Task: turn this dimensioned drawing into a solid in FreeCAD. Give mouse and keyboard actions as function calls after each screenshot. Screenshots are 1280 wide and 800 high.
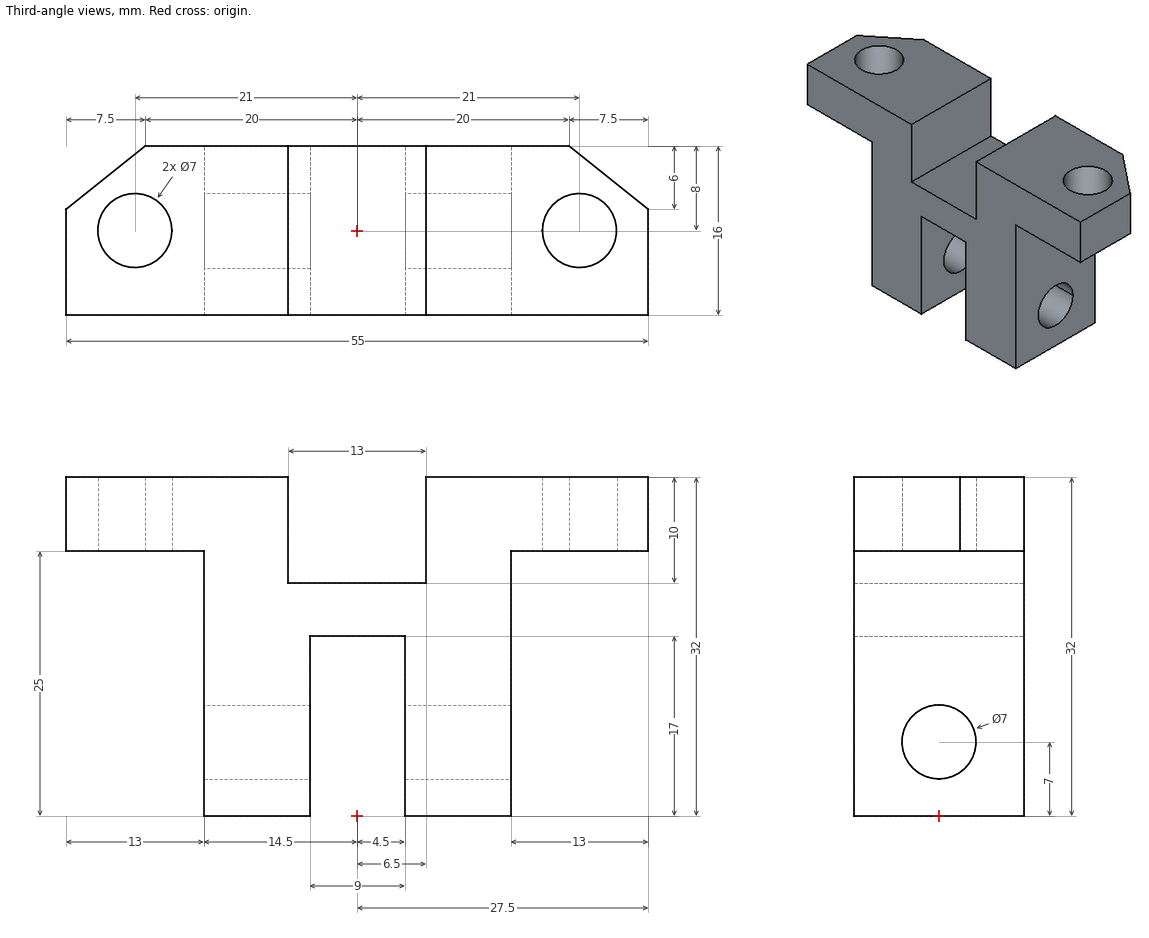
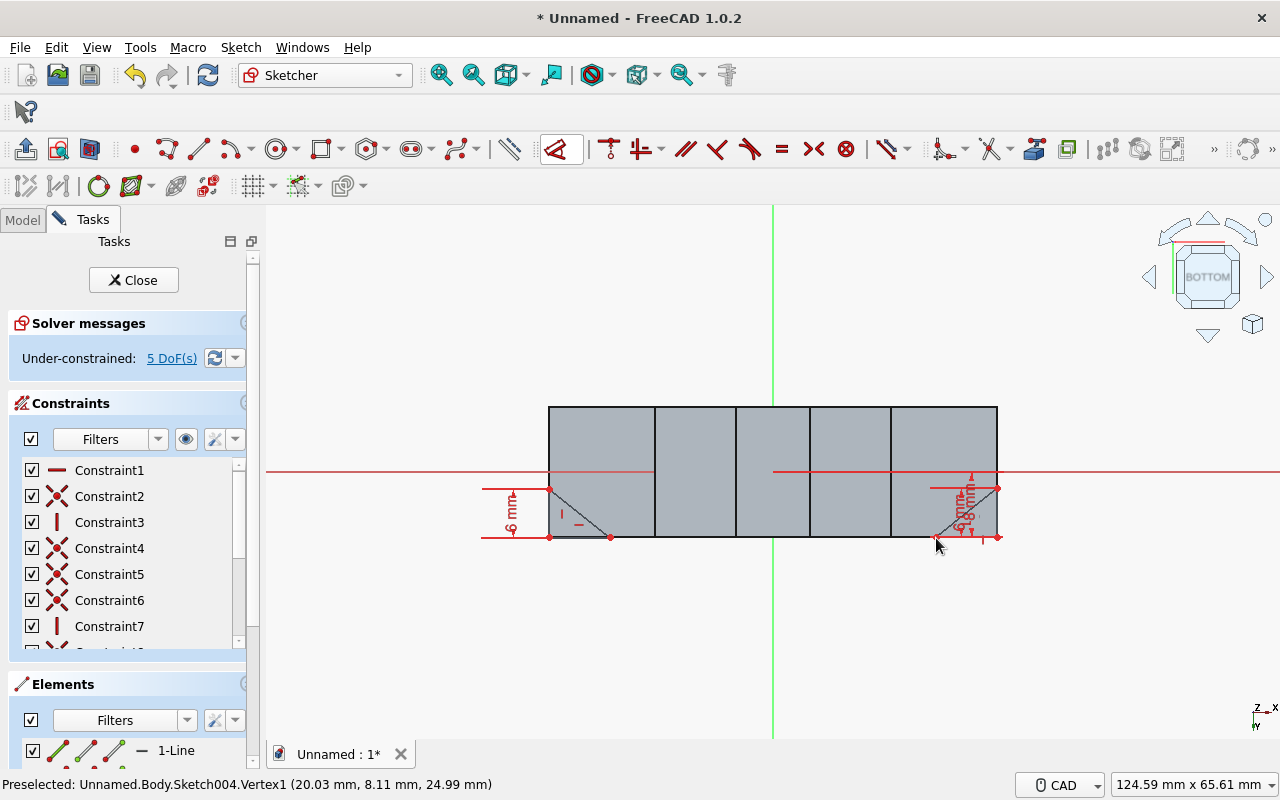
click(610, 538)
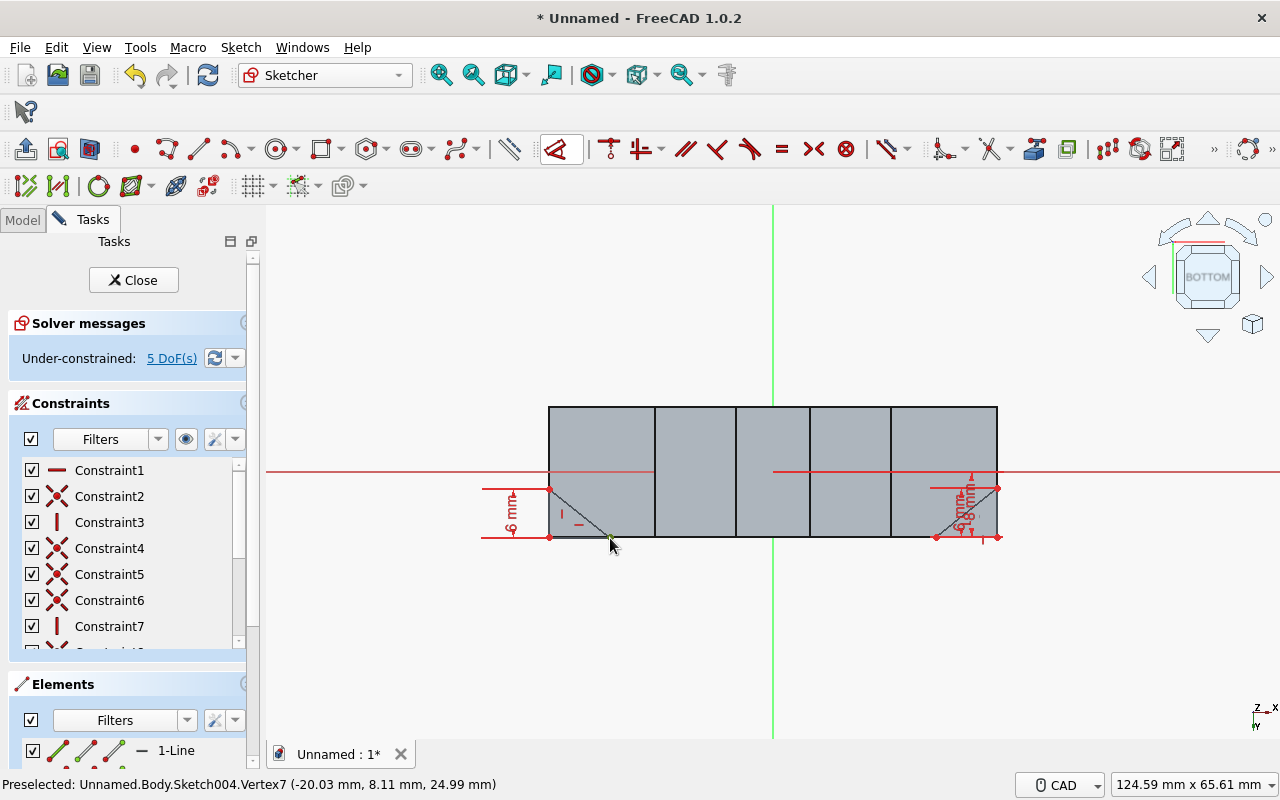
key(i)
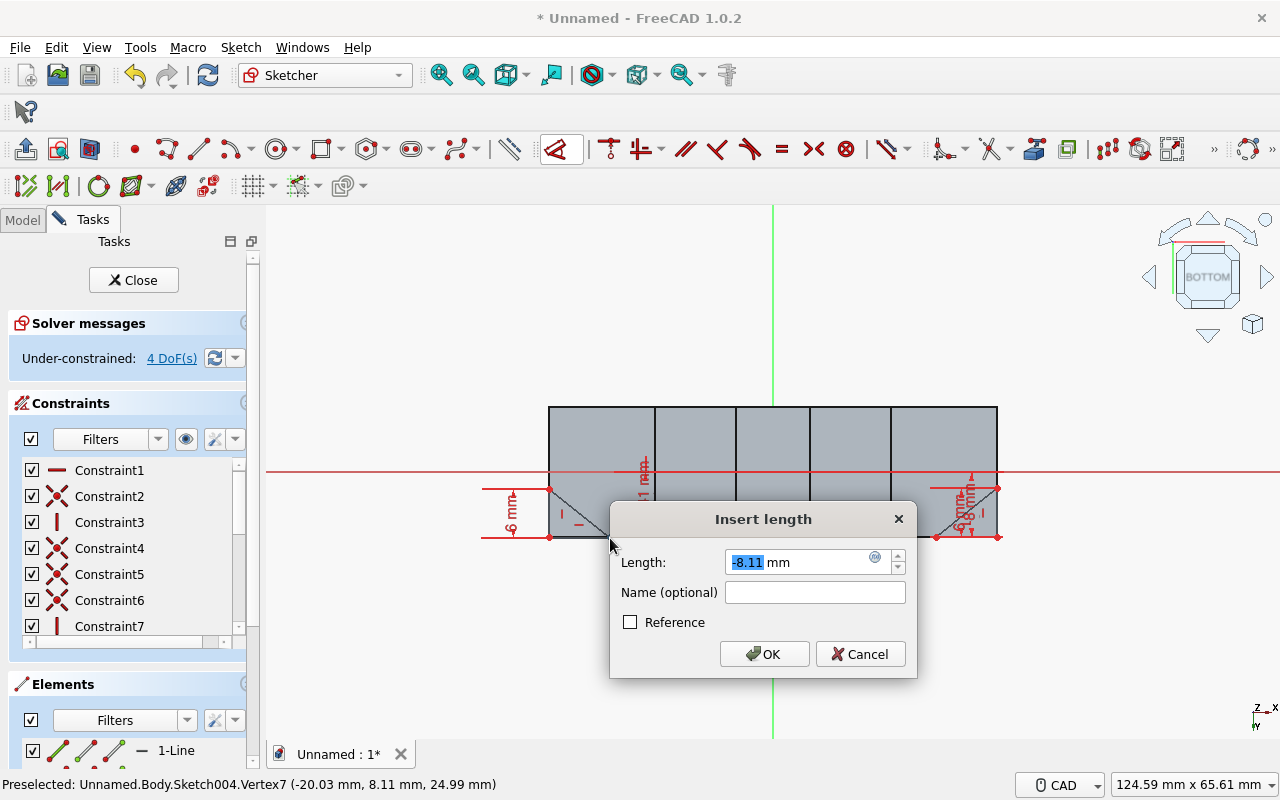
text(-8)
key(Return)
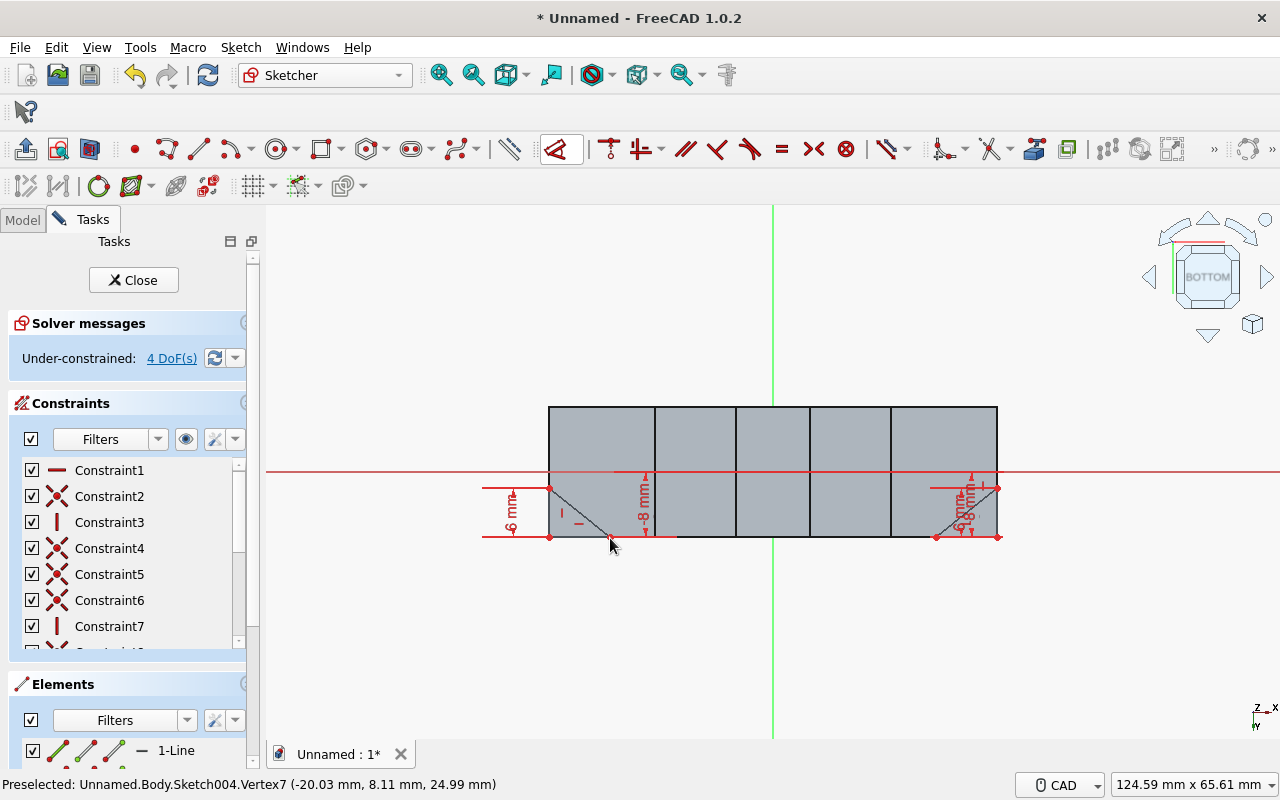
click(954, 537)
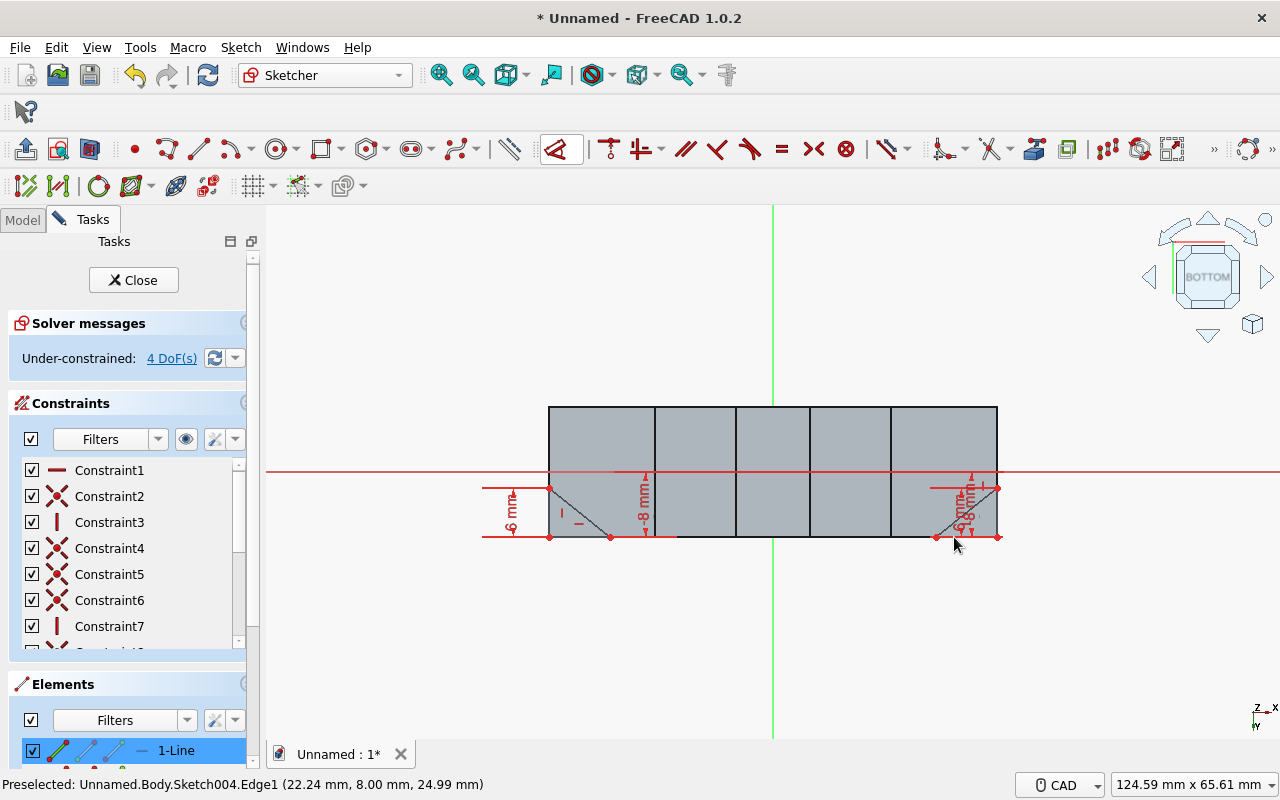
click(578, 150)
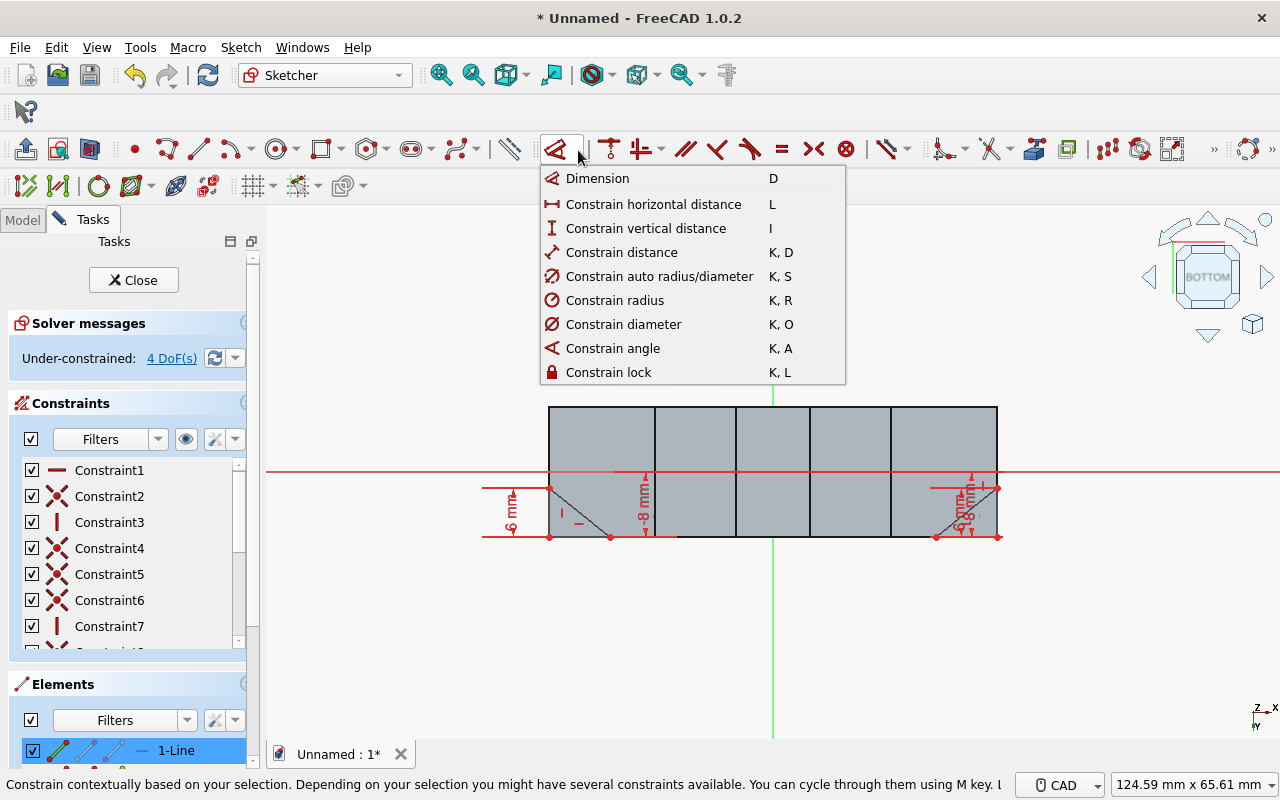
click(693, 204)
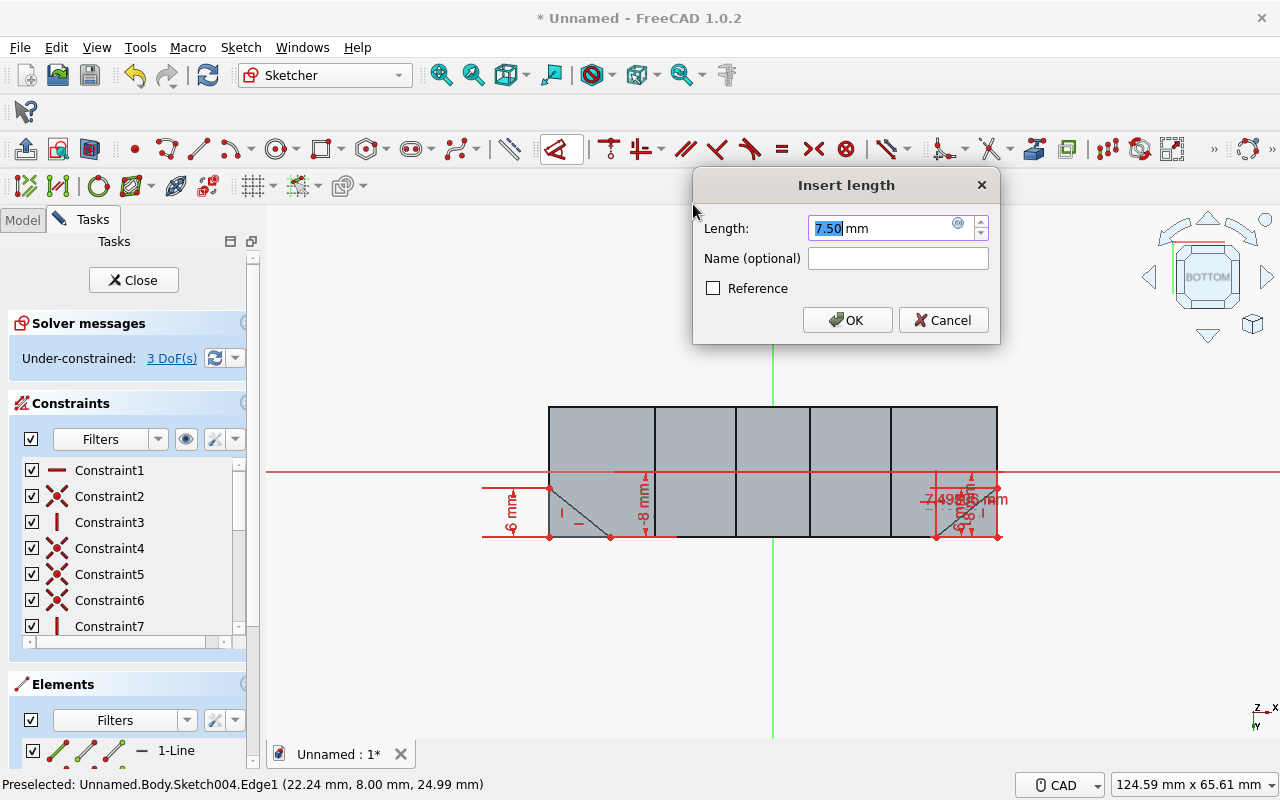
text(7.5)
key(Return)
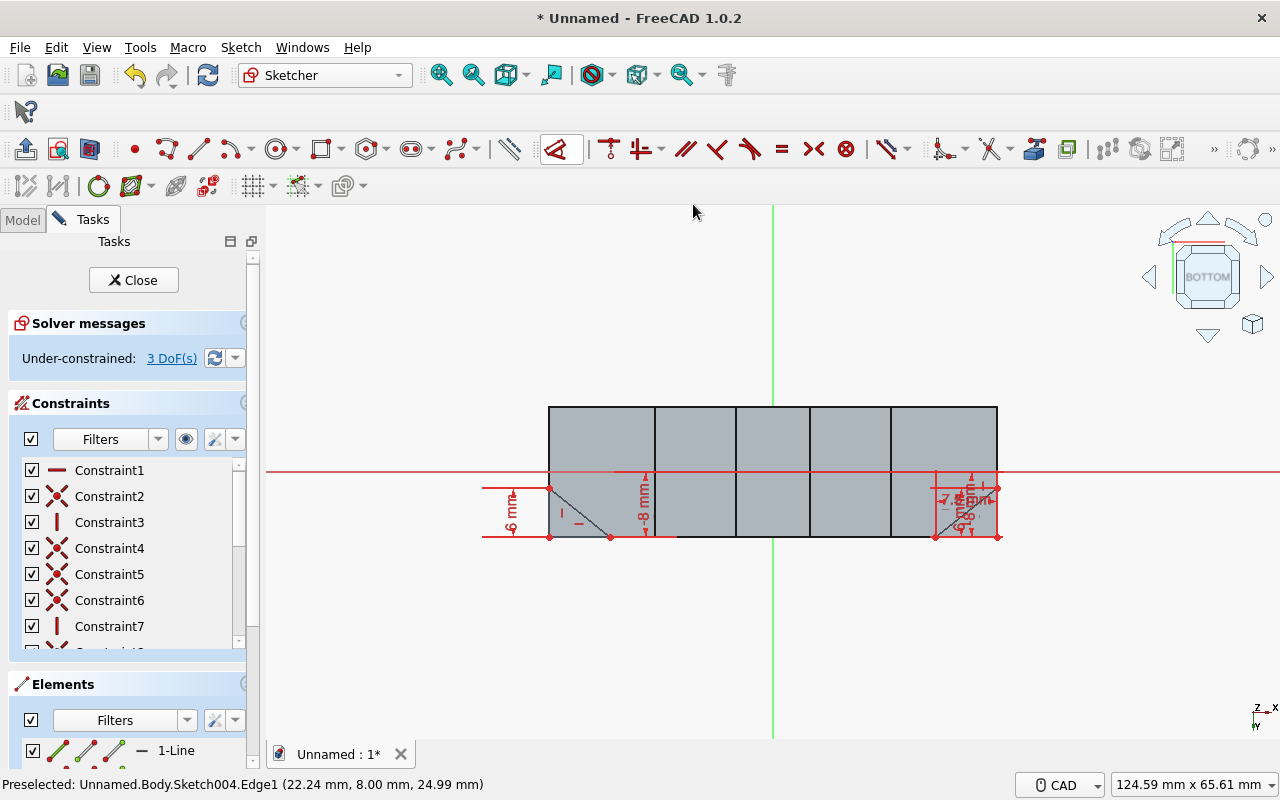
click(567, 537)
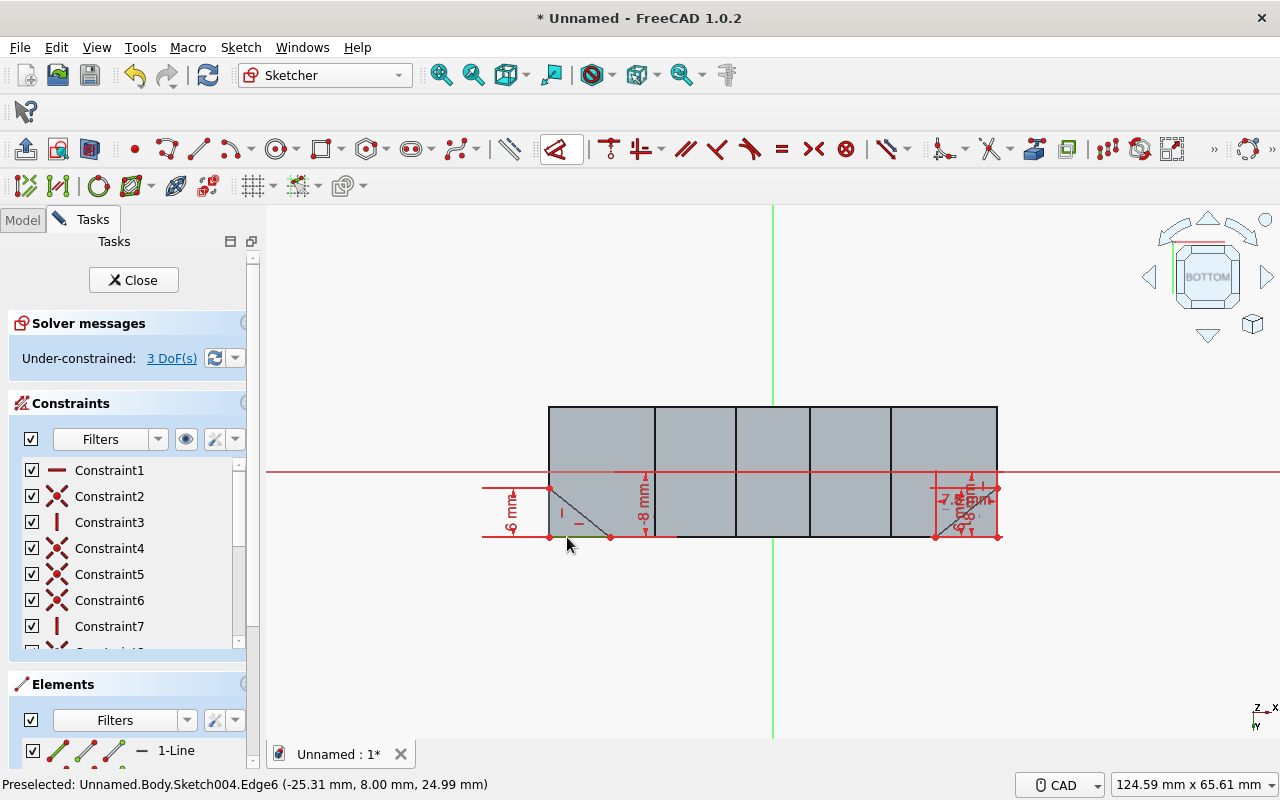
key(l)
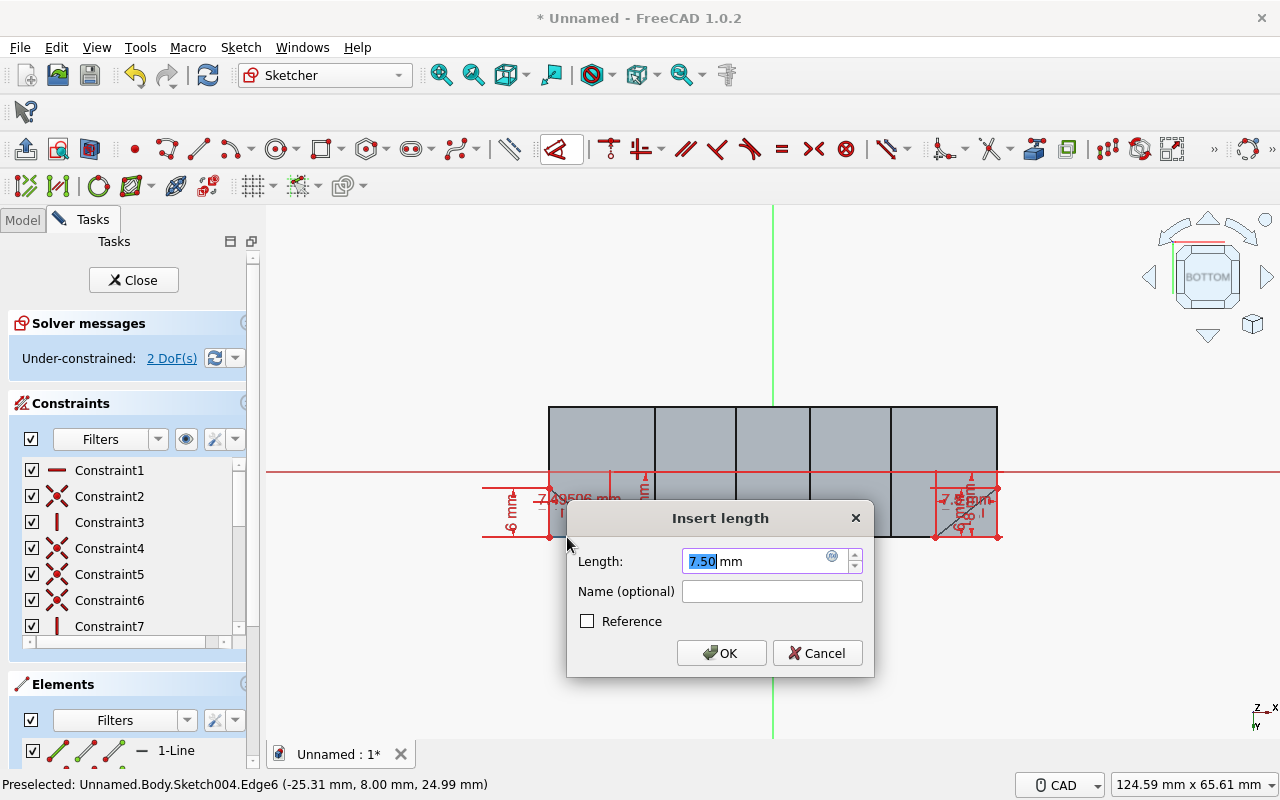
text(7.5)
key(Return)